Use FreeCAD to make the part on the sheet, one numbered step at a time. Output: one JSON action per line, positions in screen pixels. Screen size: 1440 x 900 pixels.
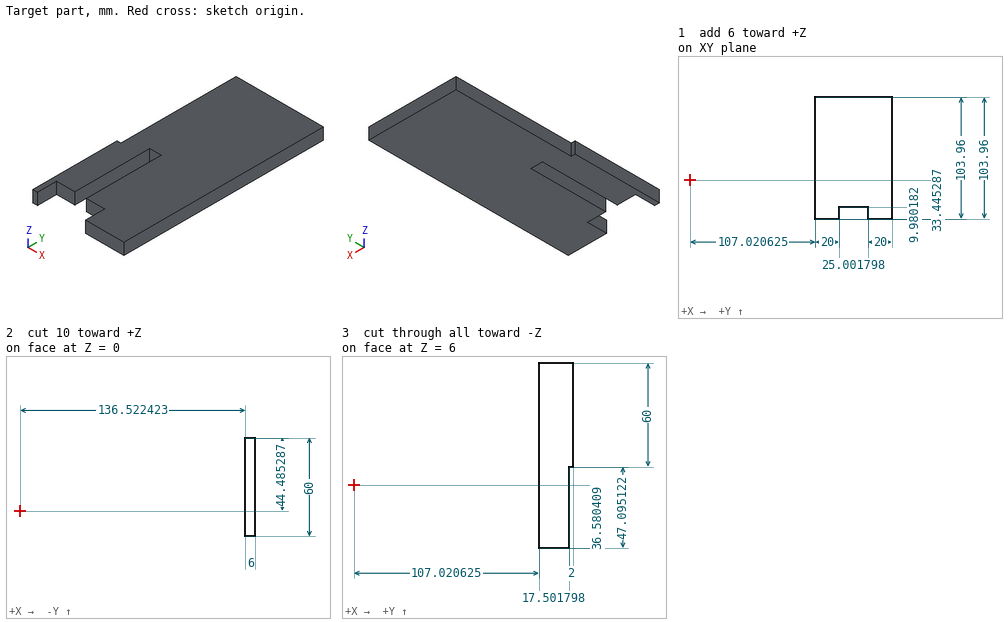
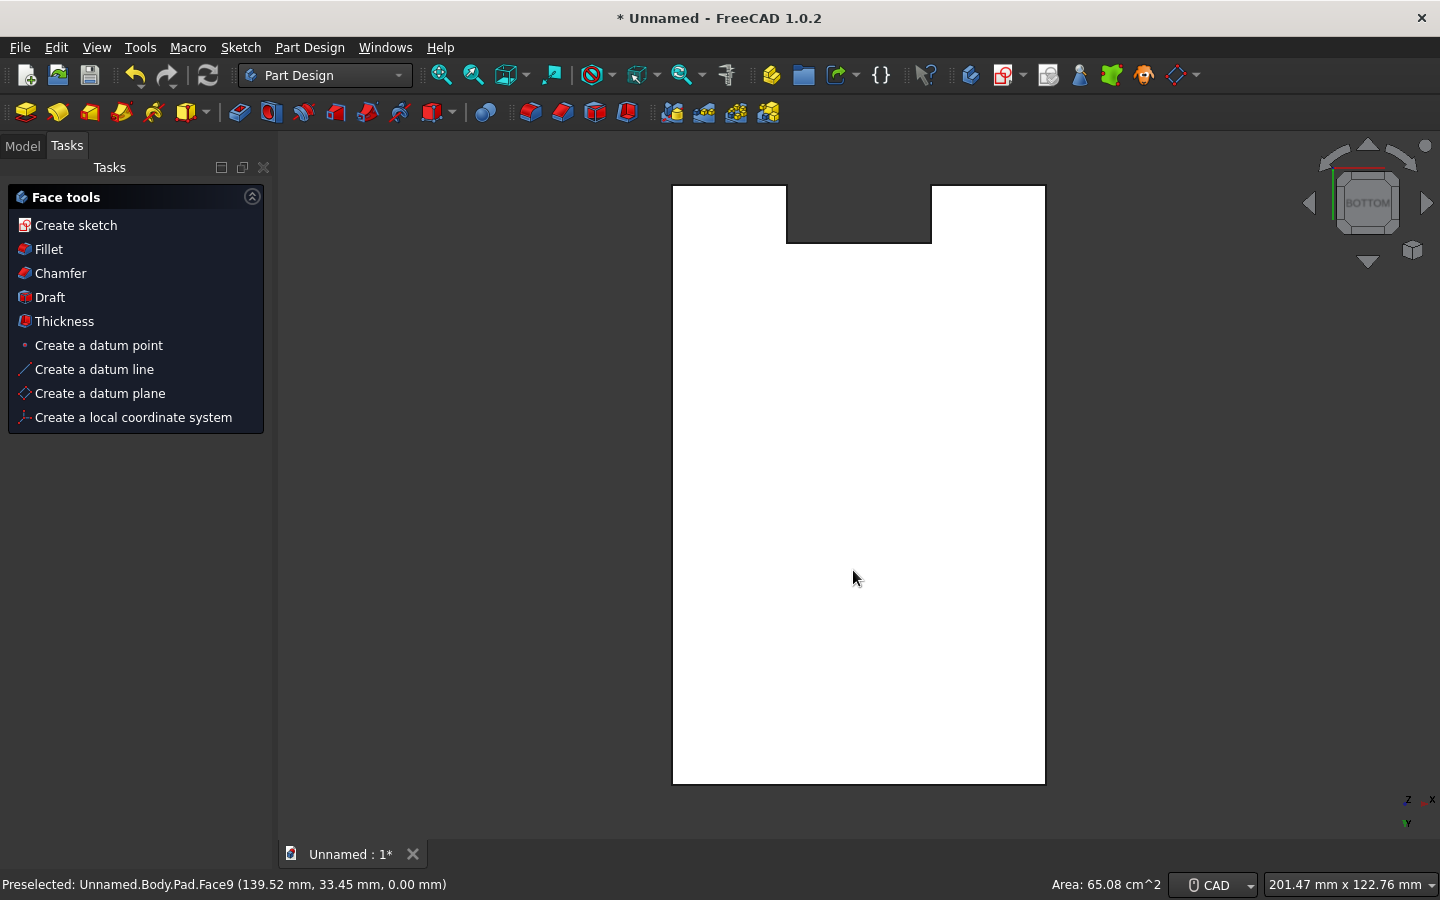
{"action": "left_click", "coordinate": [1004, 76]}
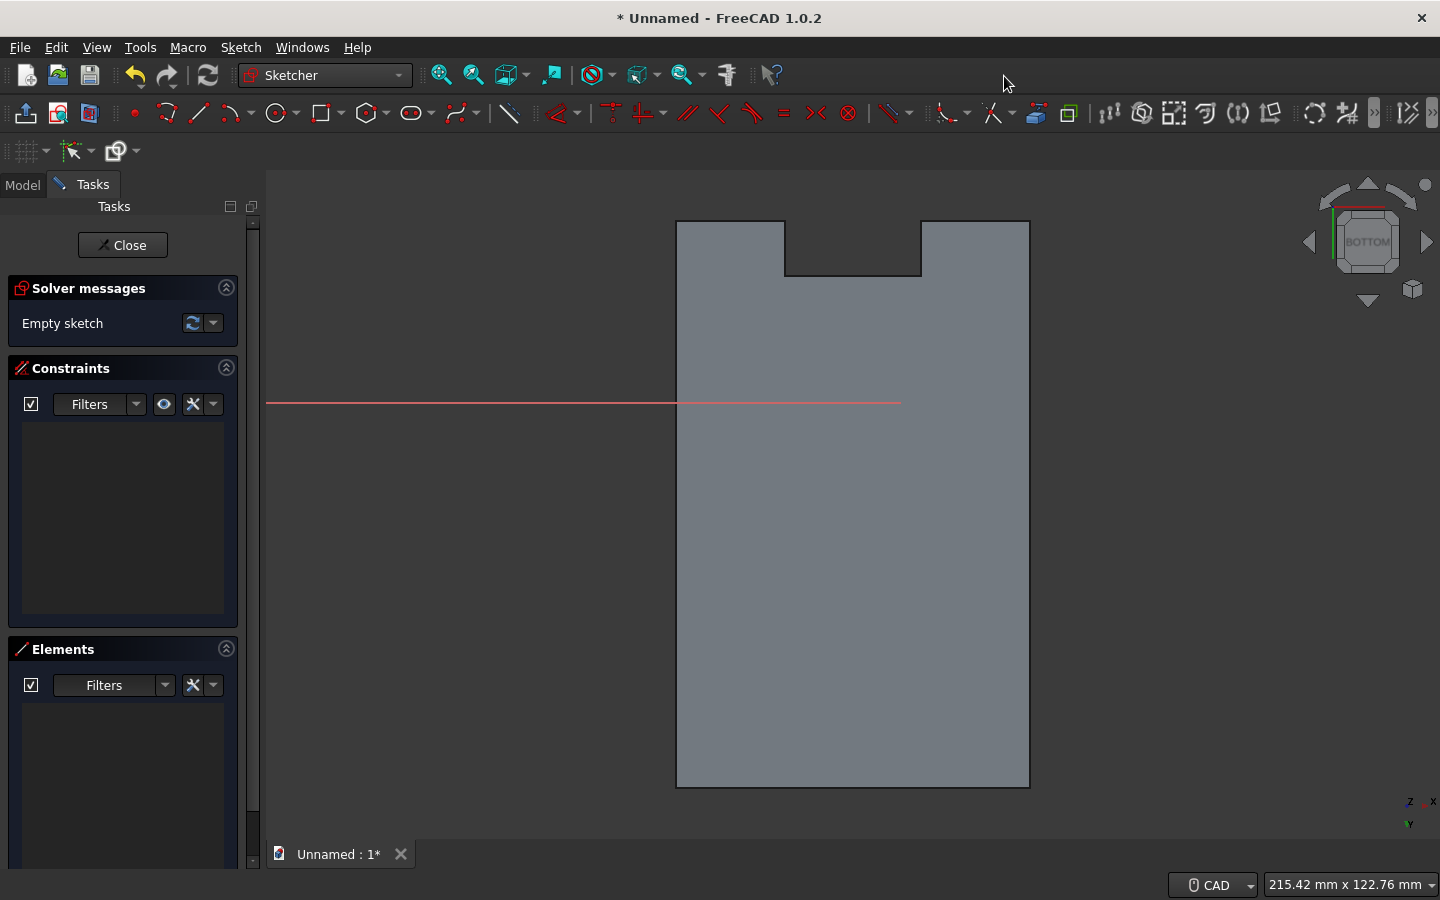
{"action": "scroll", "coordinate": [1275, 811], "scroll_direction": "down", "scroll_amount": 2}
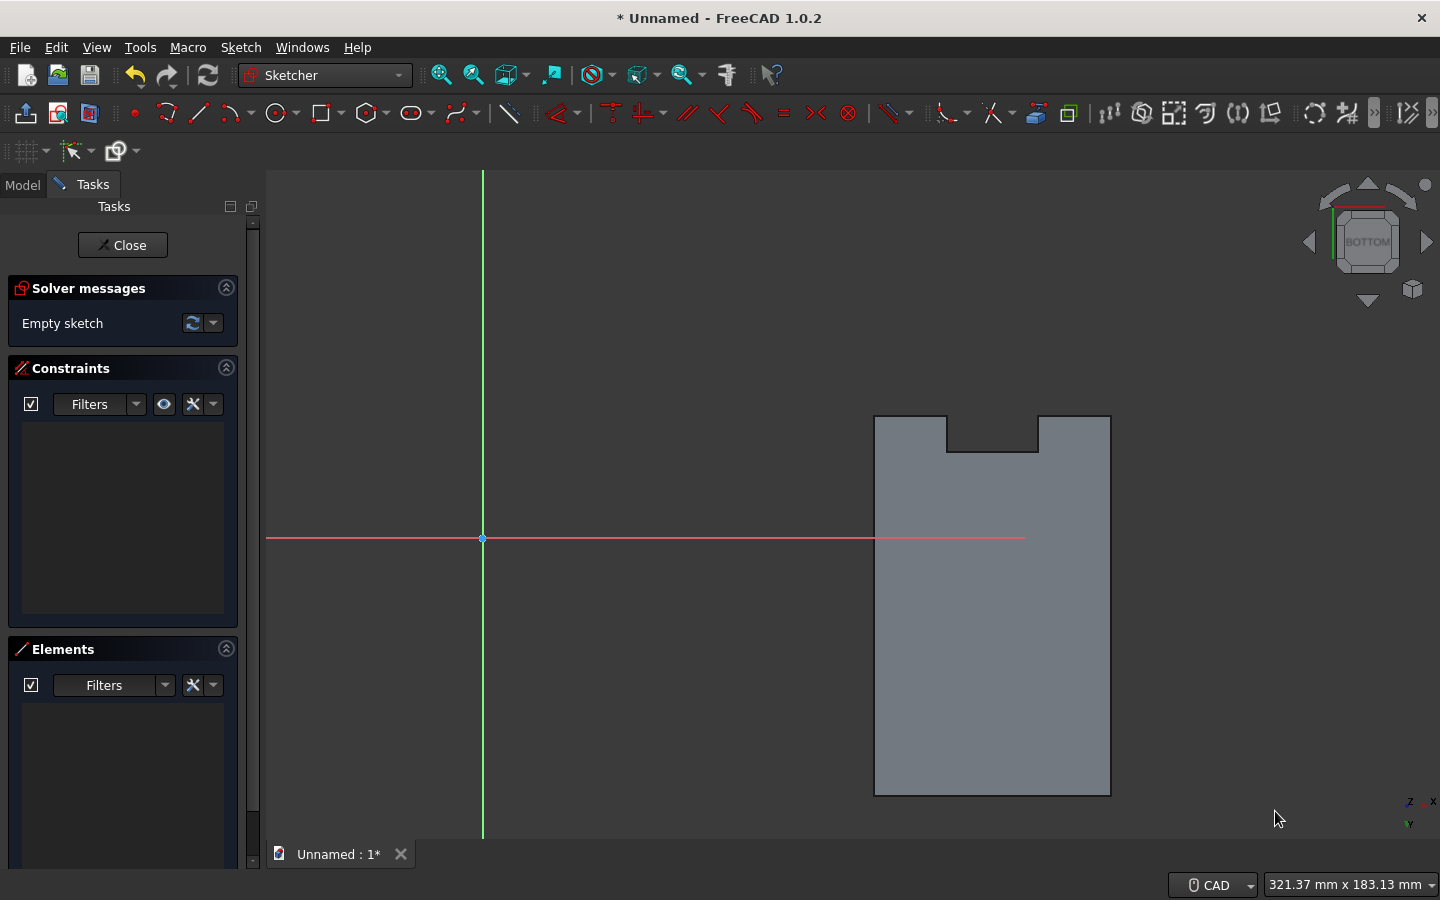
{"action": "left_click", "coordinate": [322, 114]}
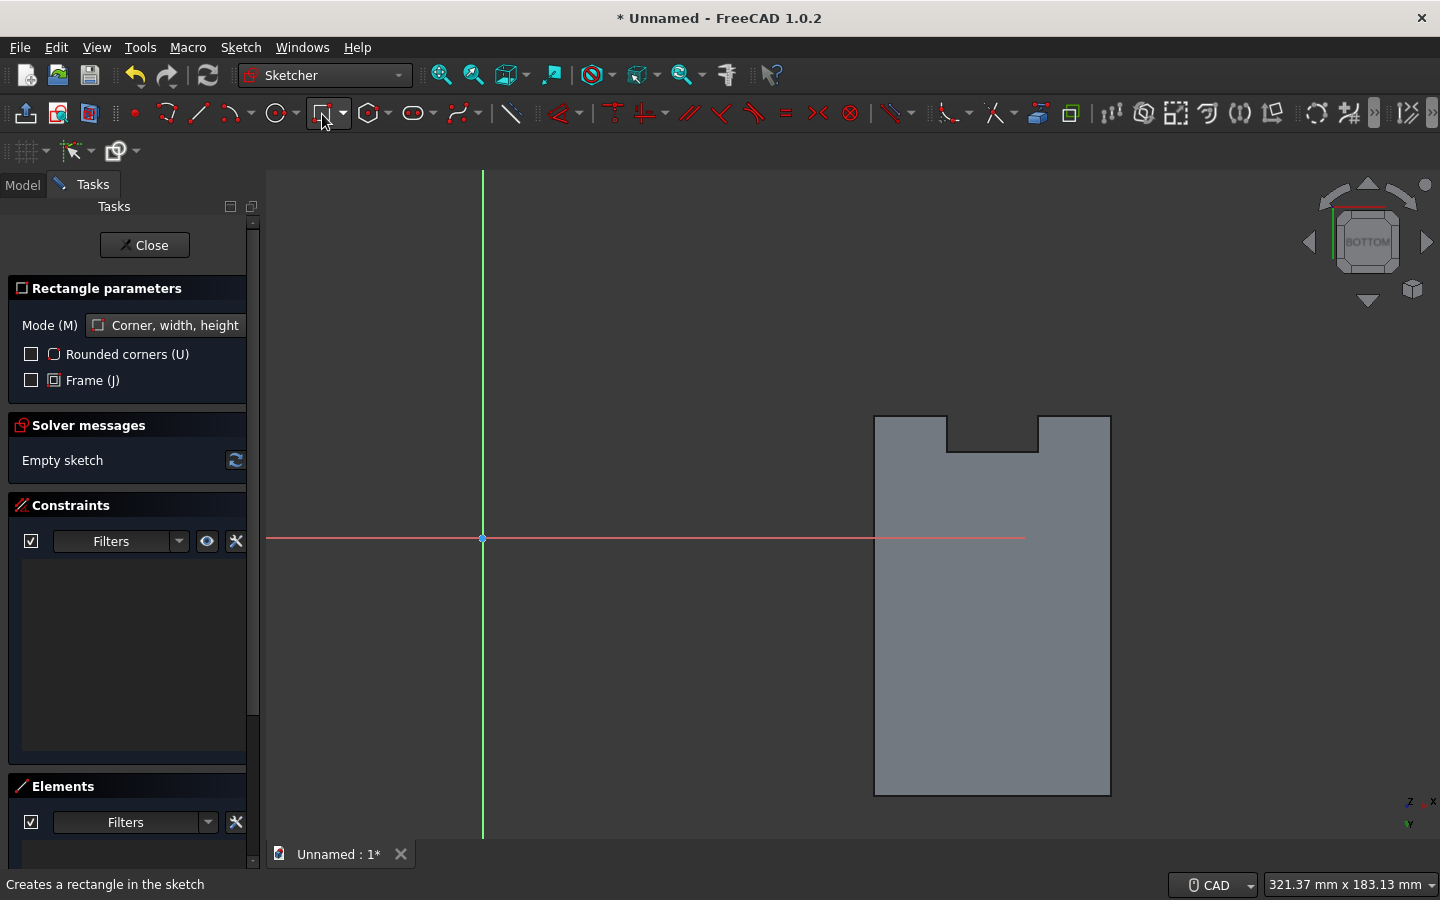
{"action": "left_click", "coordinate": [981, 376]}
{"action": "left_click", "coordinate": [1003, 595]}
{"action": "key", "text": "Escape"}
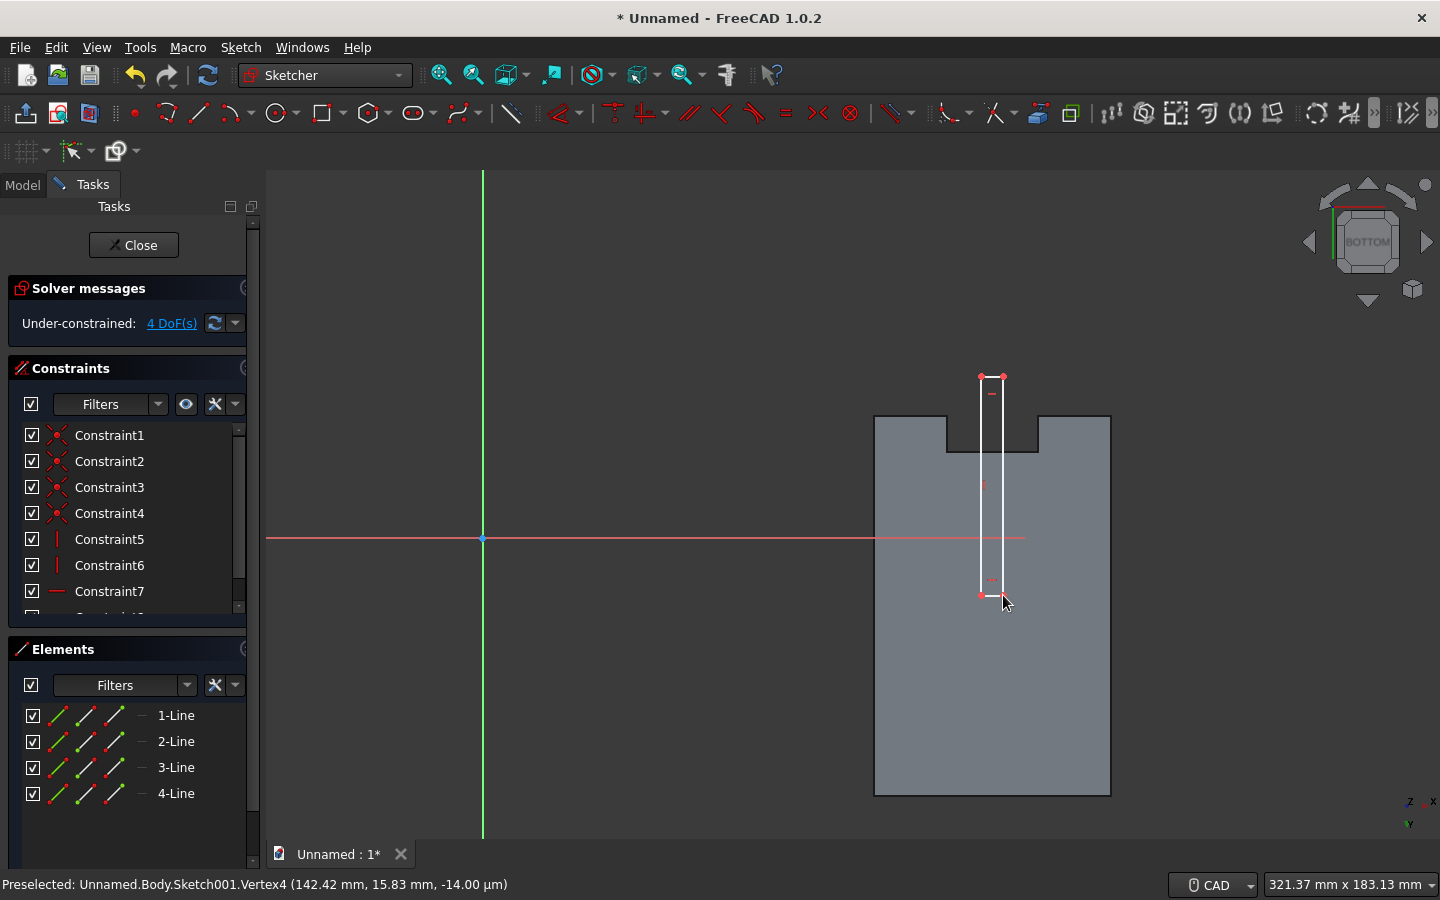
{"action": "key", "text": "d"}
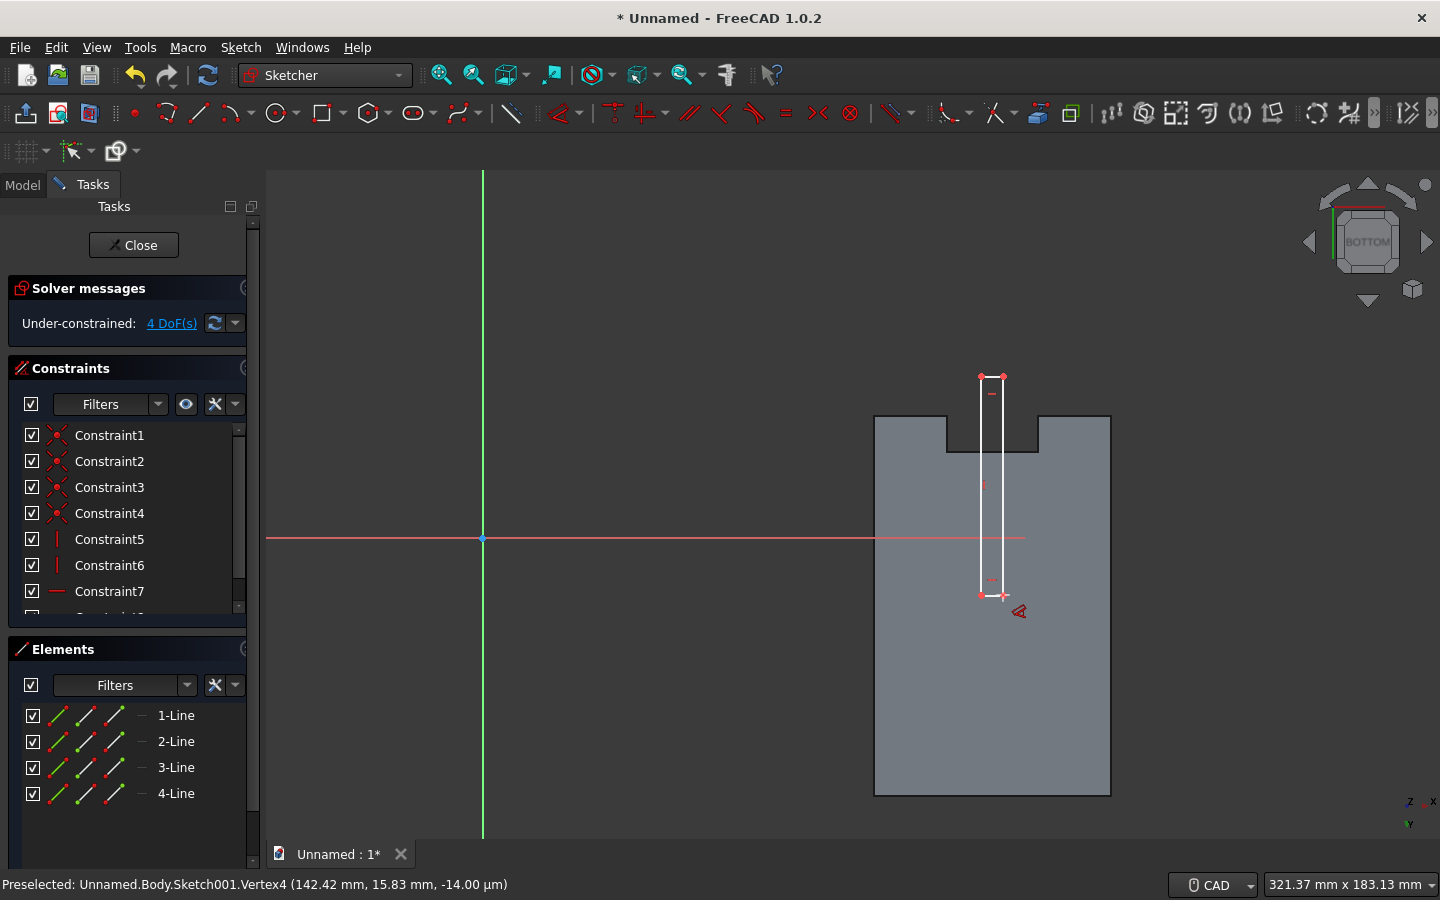
{"action": "scroll", "coordinate": [992, 596], "scroll_direction": "up", "scroll_amount": 3}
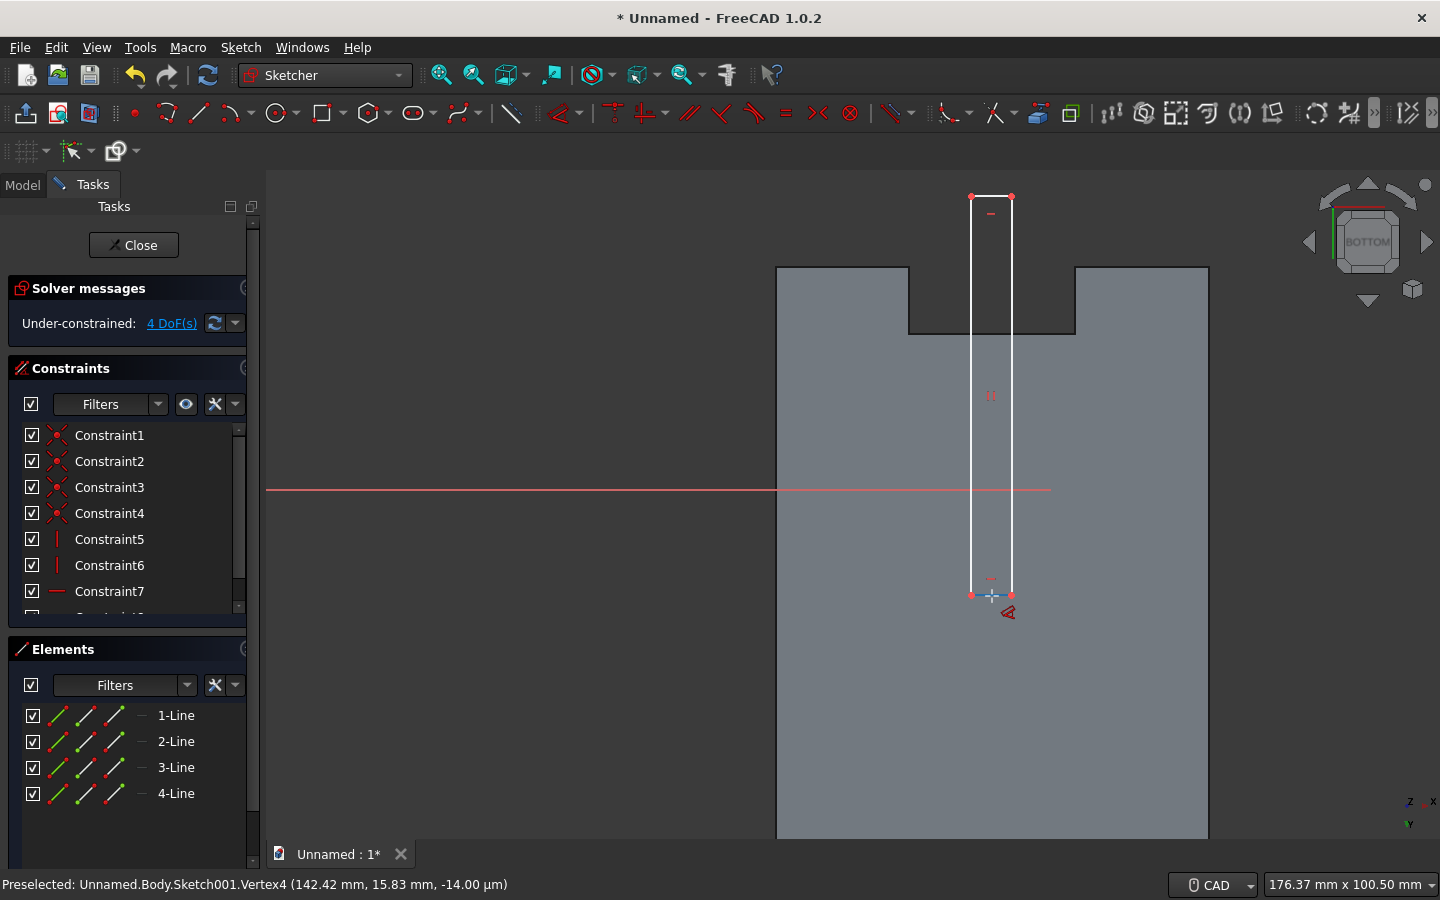
{"action": "left_click", "coordinate": [991, 595]}
{"action": "left_click", "coordinate": [991, 629]}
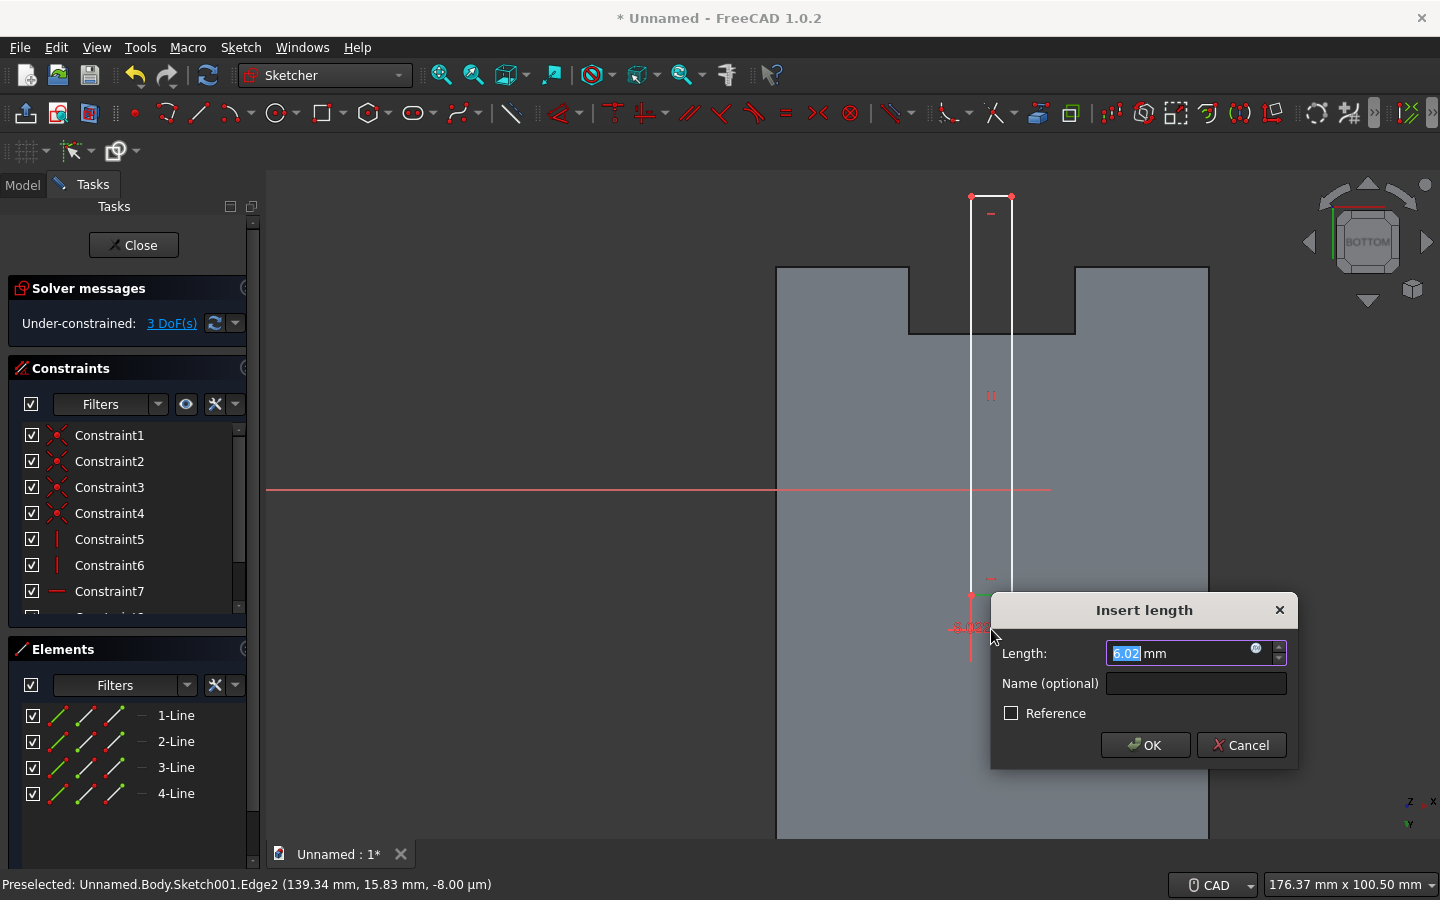
{"action": "type", "text": "6"}
{"action": "key", "text": "Return"}